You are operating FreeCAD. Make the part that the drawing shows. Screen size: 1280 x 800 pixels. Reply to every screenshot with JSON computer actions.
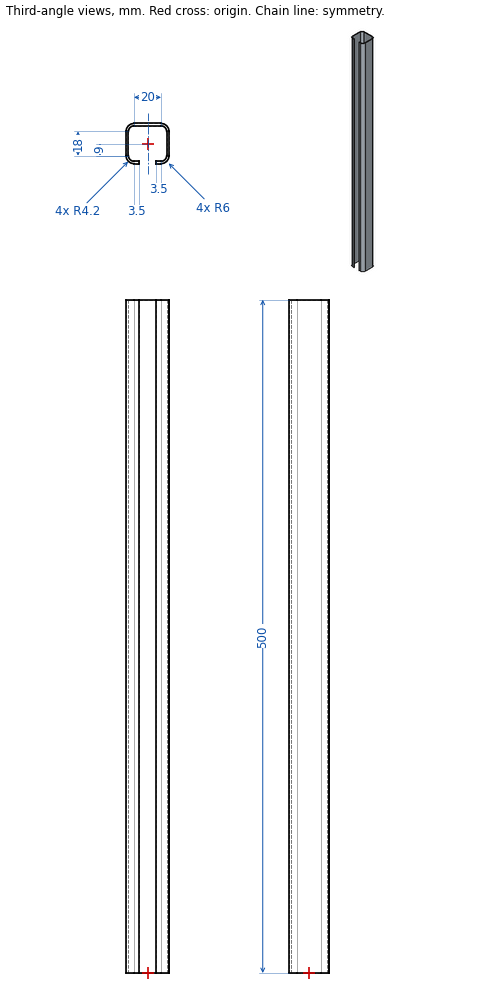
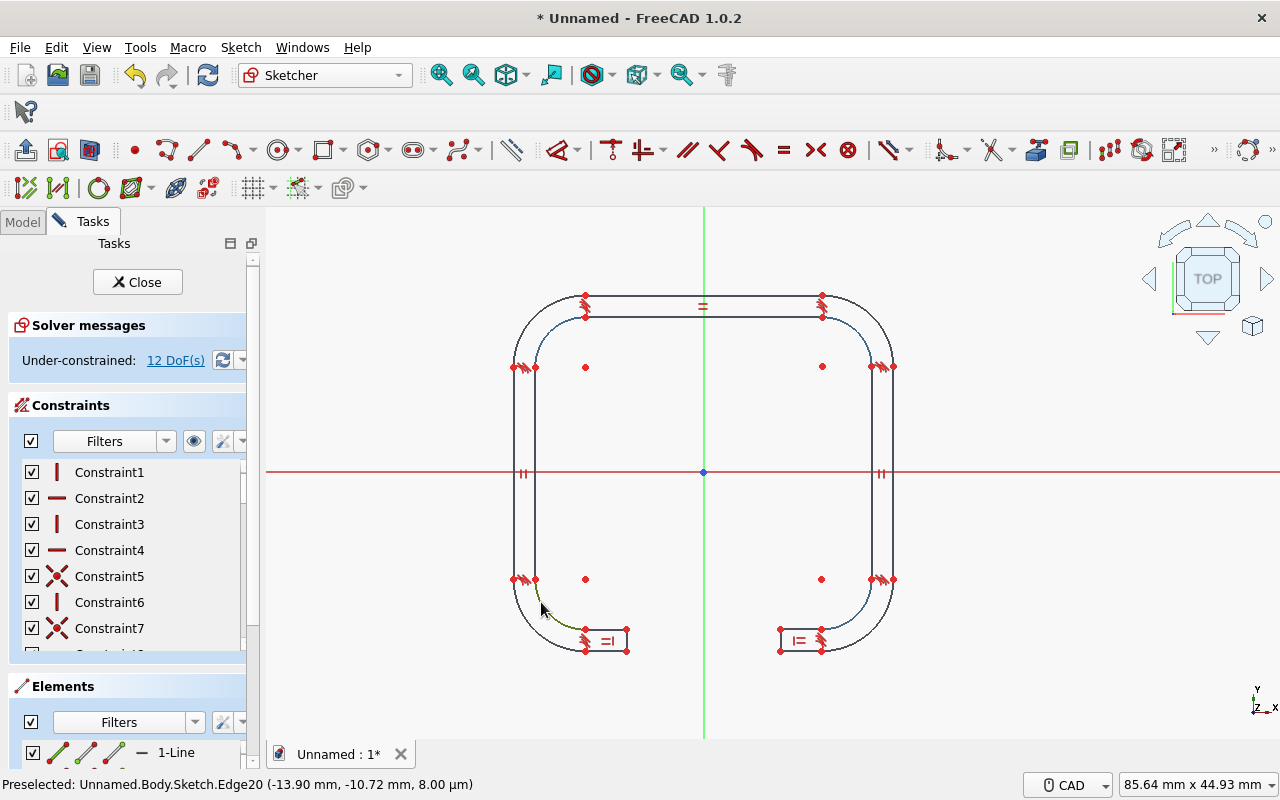
{"action": "left_click", "coordinate": [784, 150]}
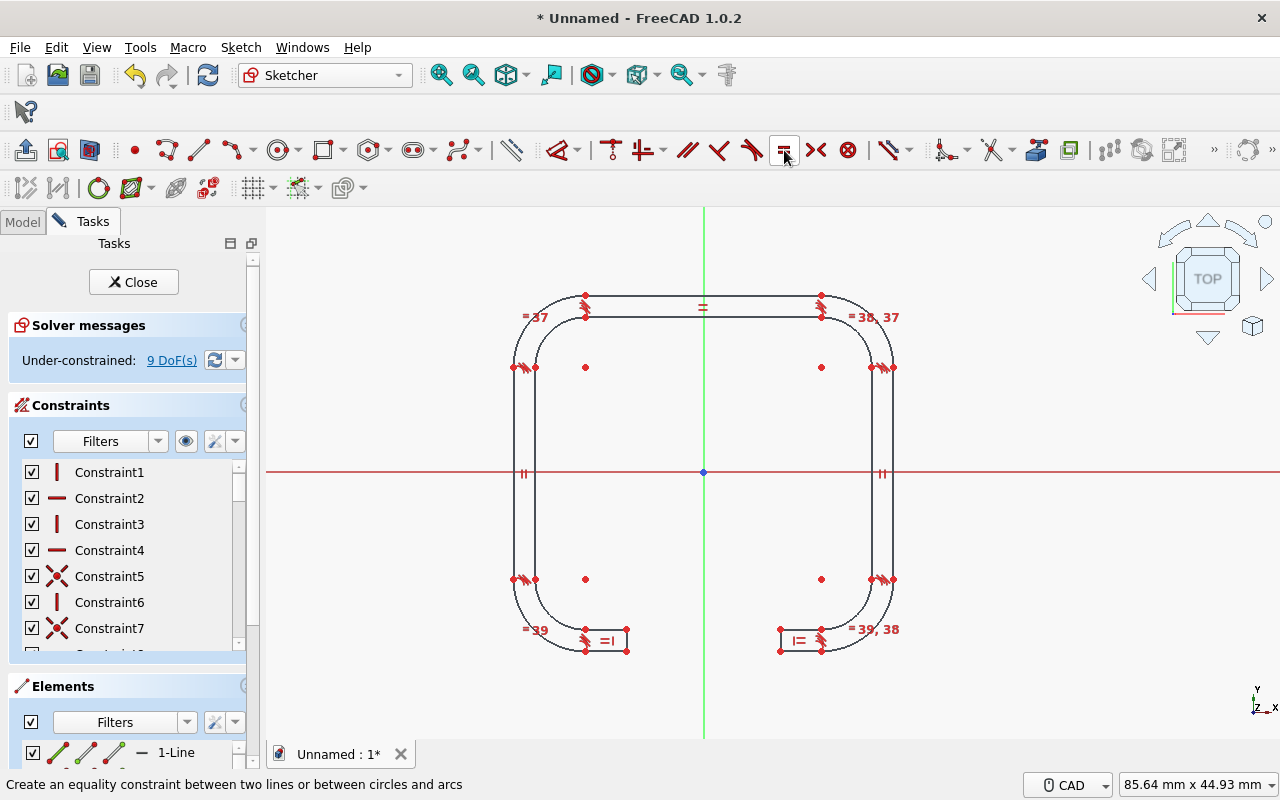
{"action": "left_click", "coordinate": [822, 580]}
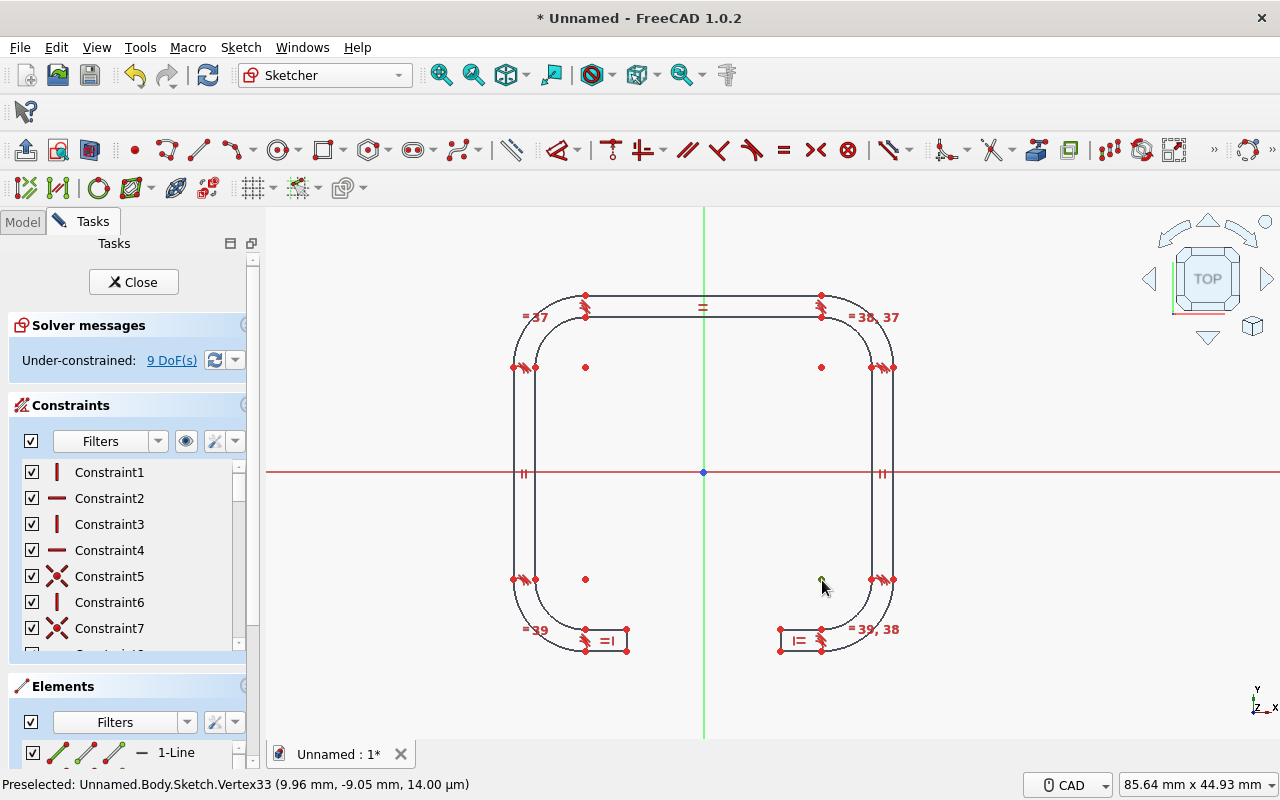
{"action": "left_click", "coordinate": [585, 580]}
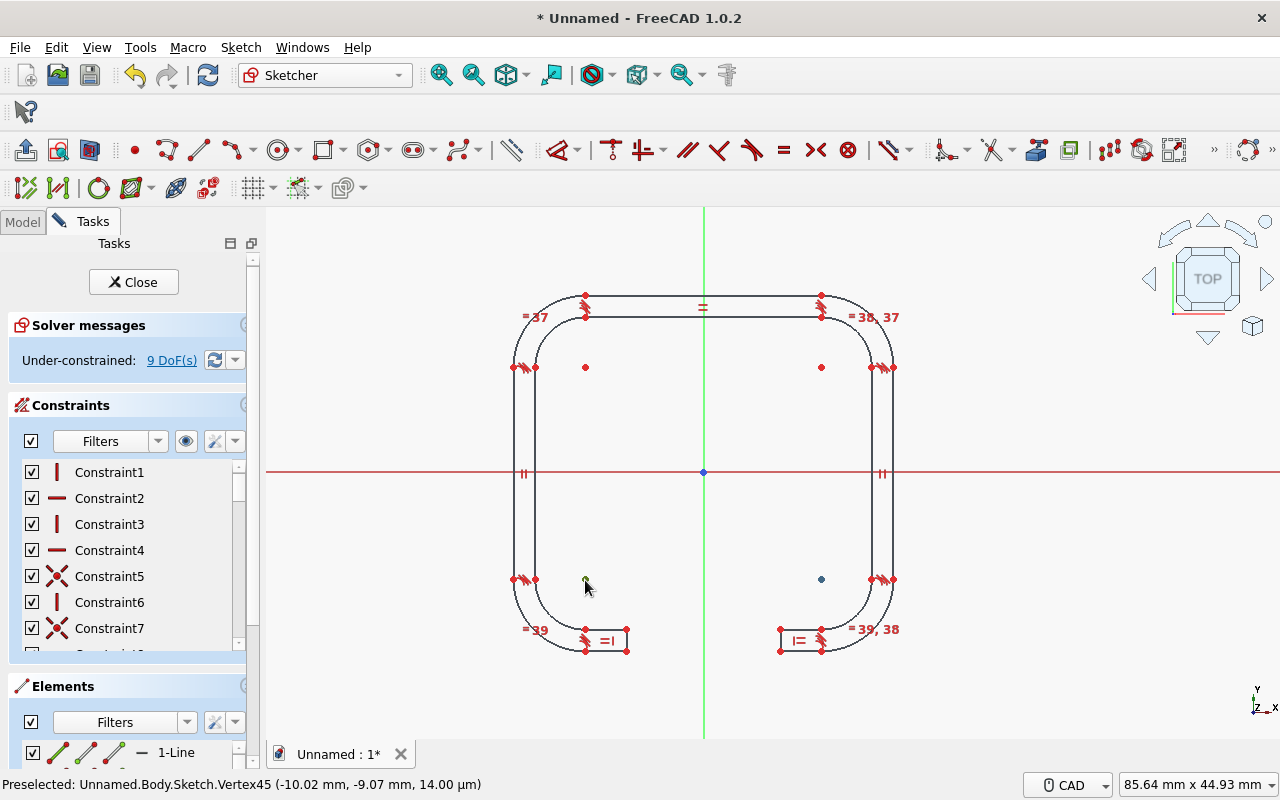
{"action": "left_click", "coordinate": [704, 677]}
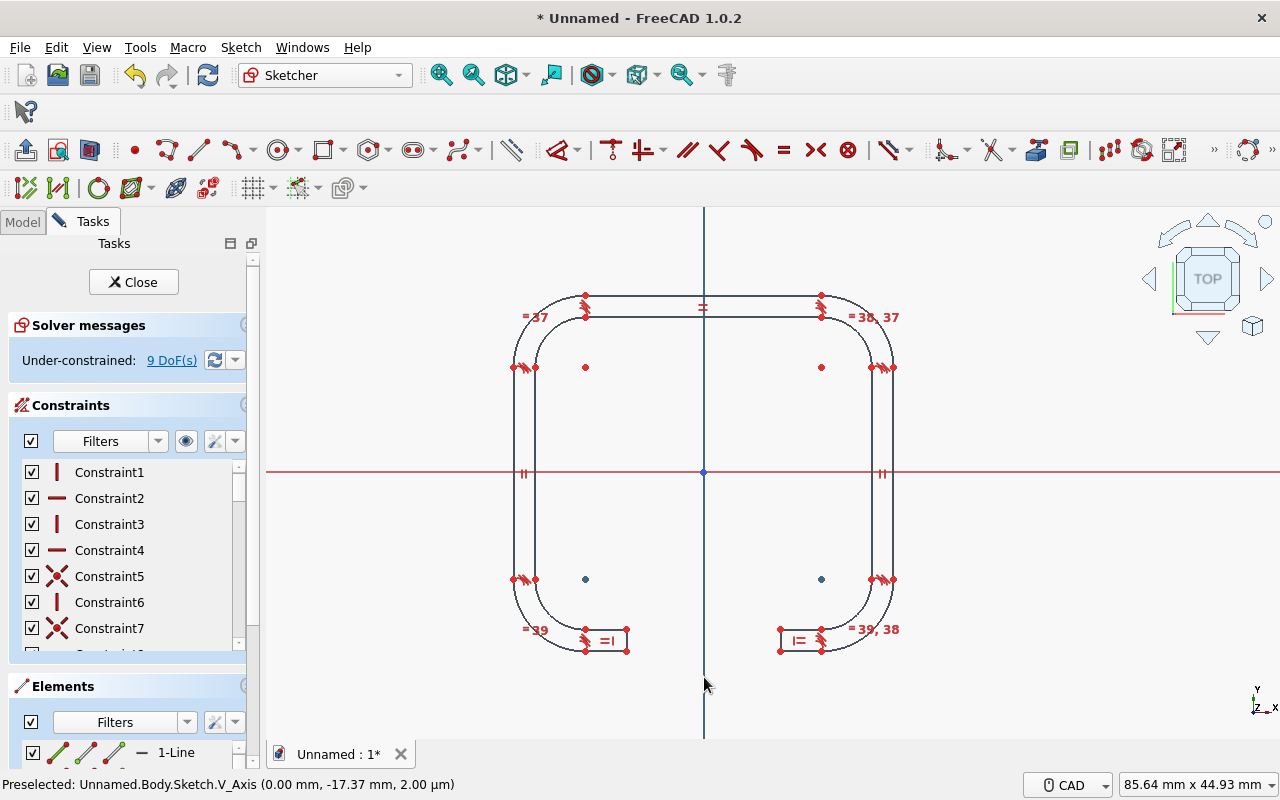
{"action": "left_click", "coordinate": [816, 150]}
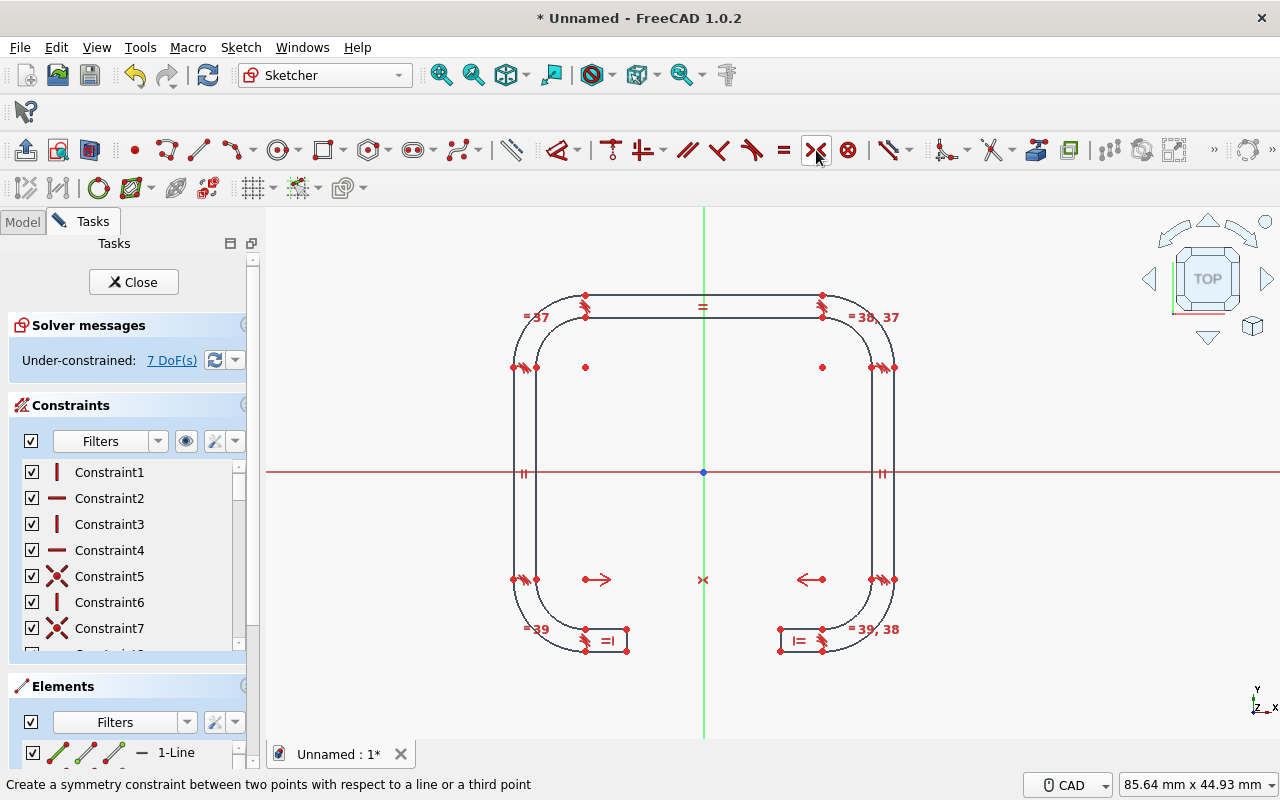
{"action": "left_click", "coordinate": [563, 323]}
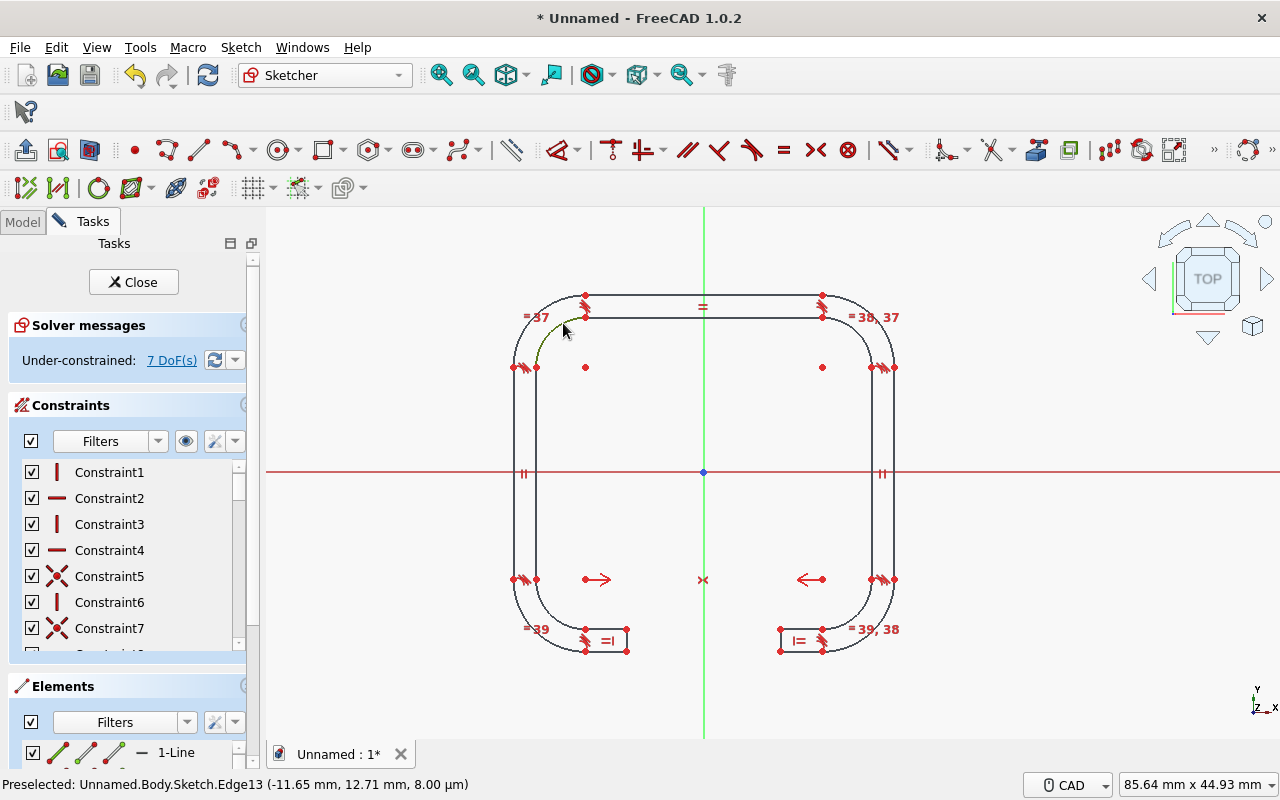
{"action": "left_click", "coordinate": [580, 150]}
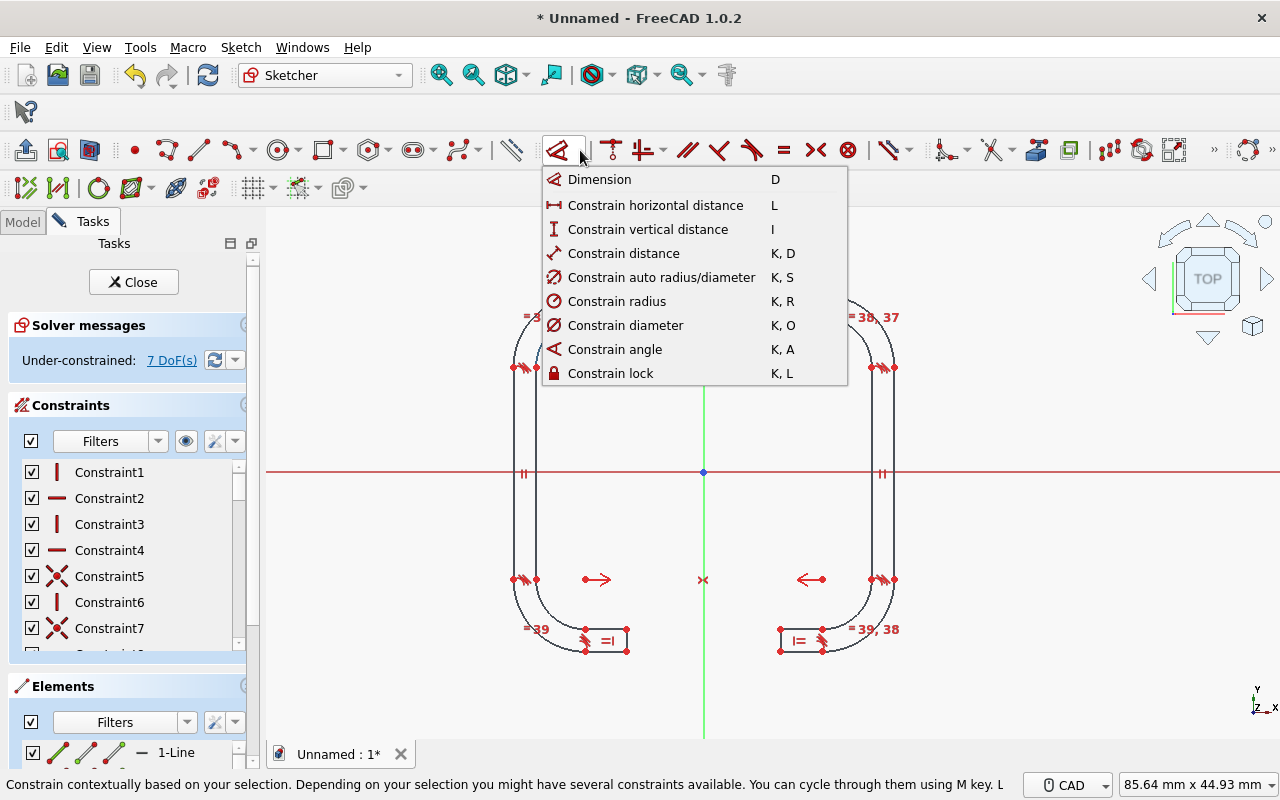
{"action": "left_click", "coordinate": [695, 301]}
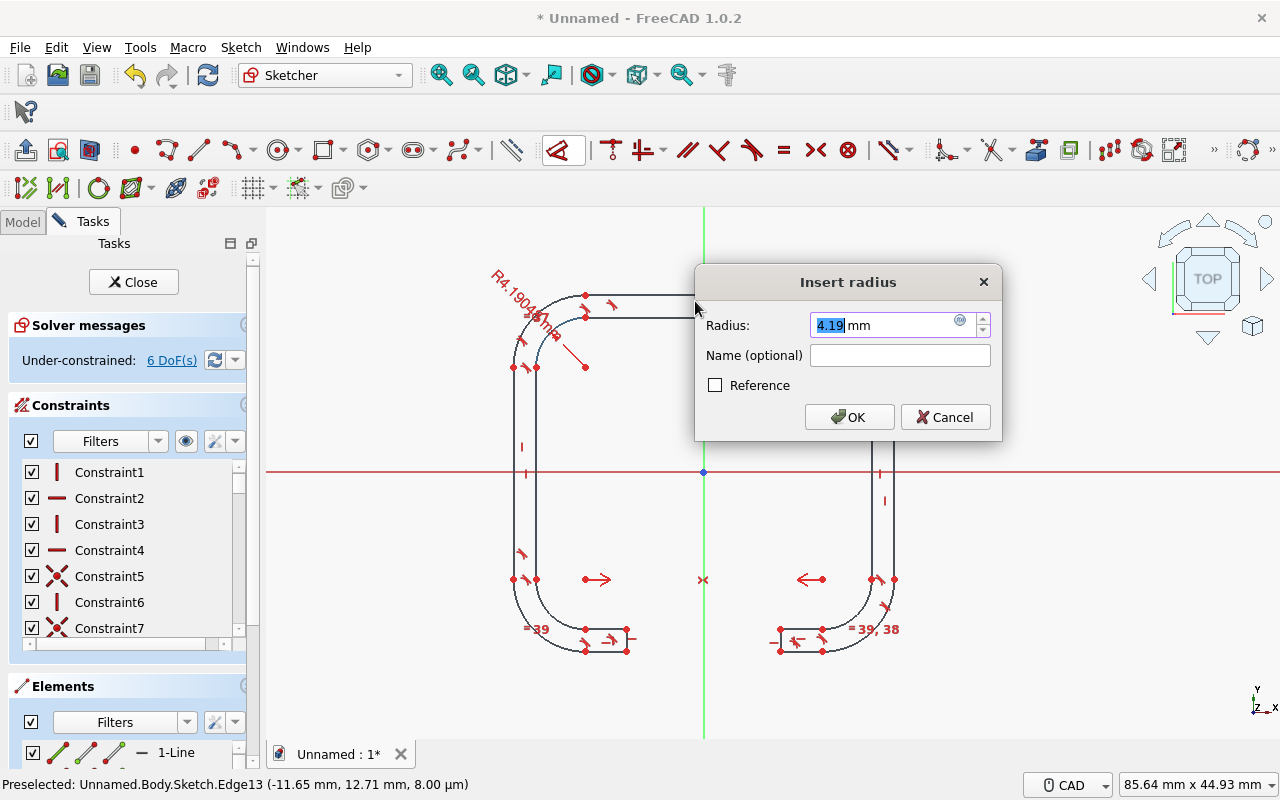
{"action": "type", "text": "4.2"}
{"action": "key", "text": "Return"}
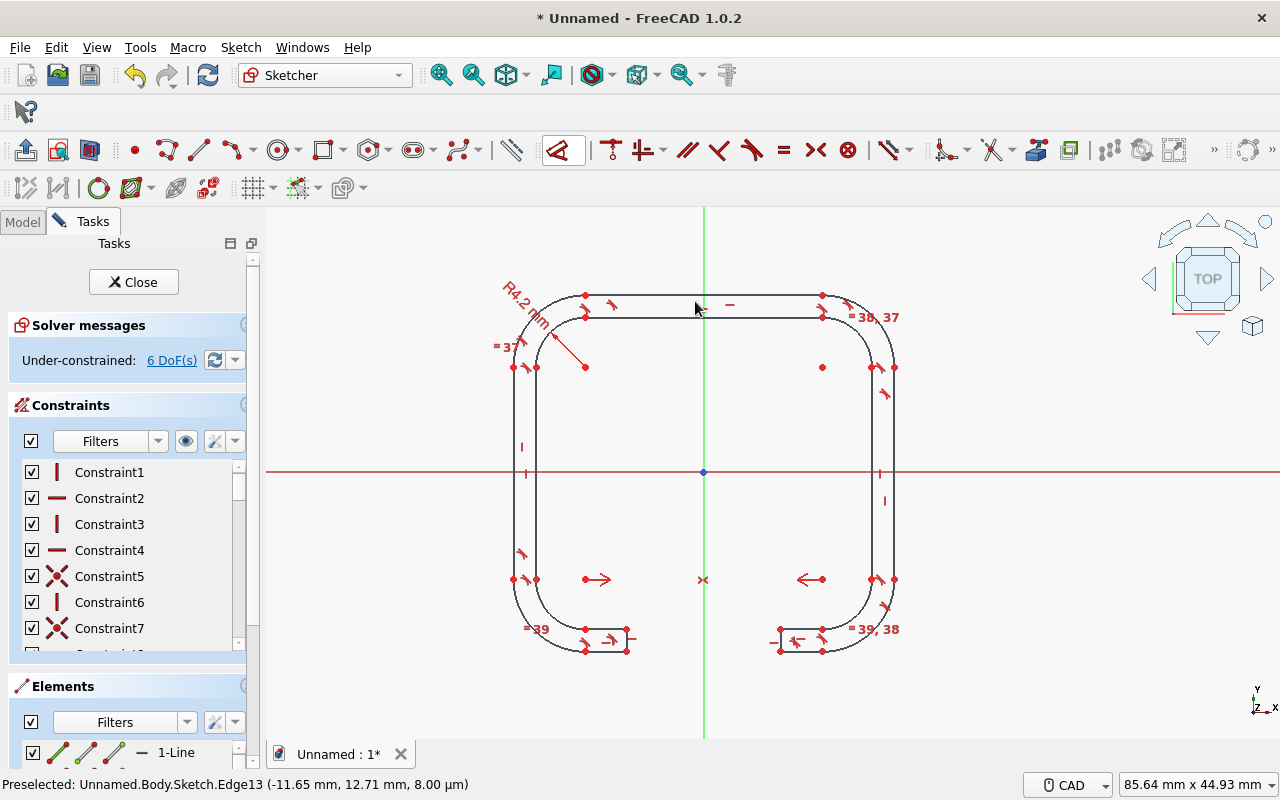
{"action": "left_click", "coordinate": [855, 644]}